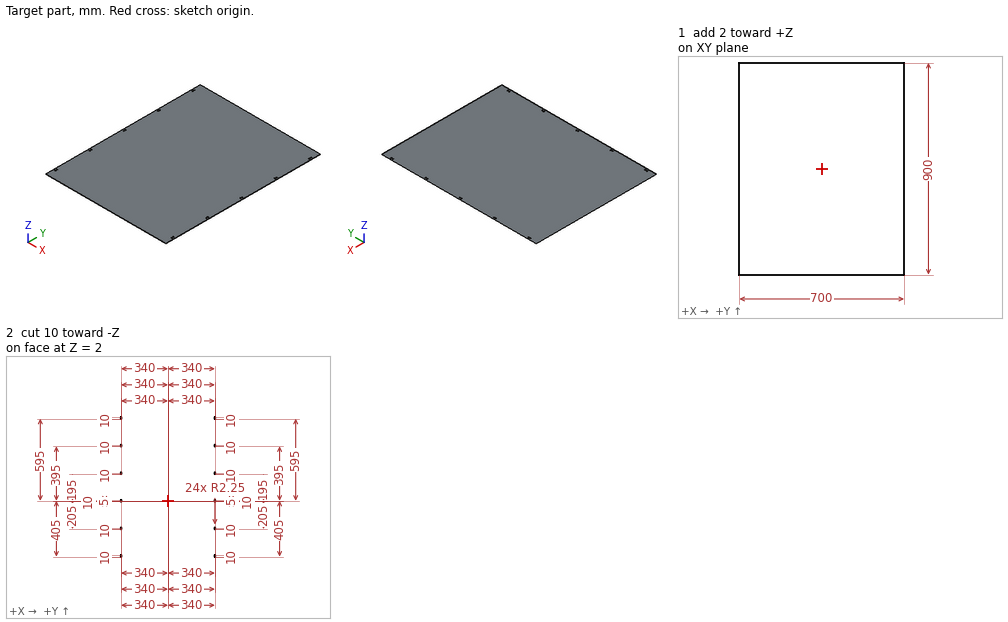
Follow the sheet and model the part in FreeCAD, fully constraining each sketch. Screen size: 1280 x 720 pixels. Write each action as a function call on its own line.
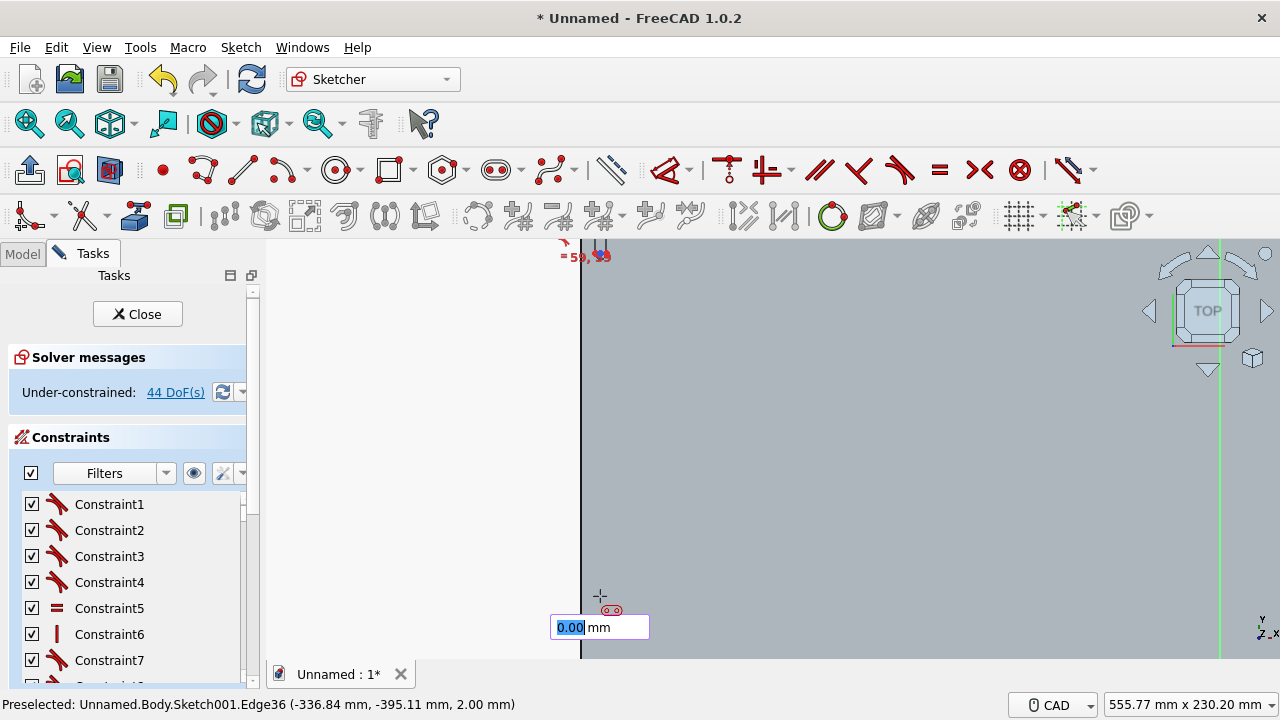
scroll(603, 606, up, 7)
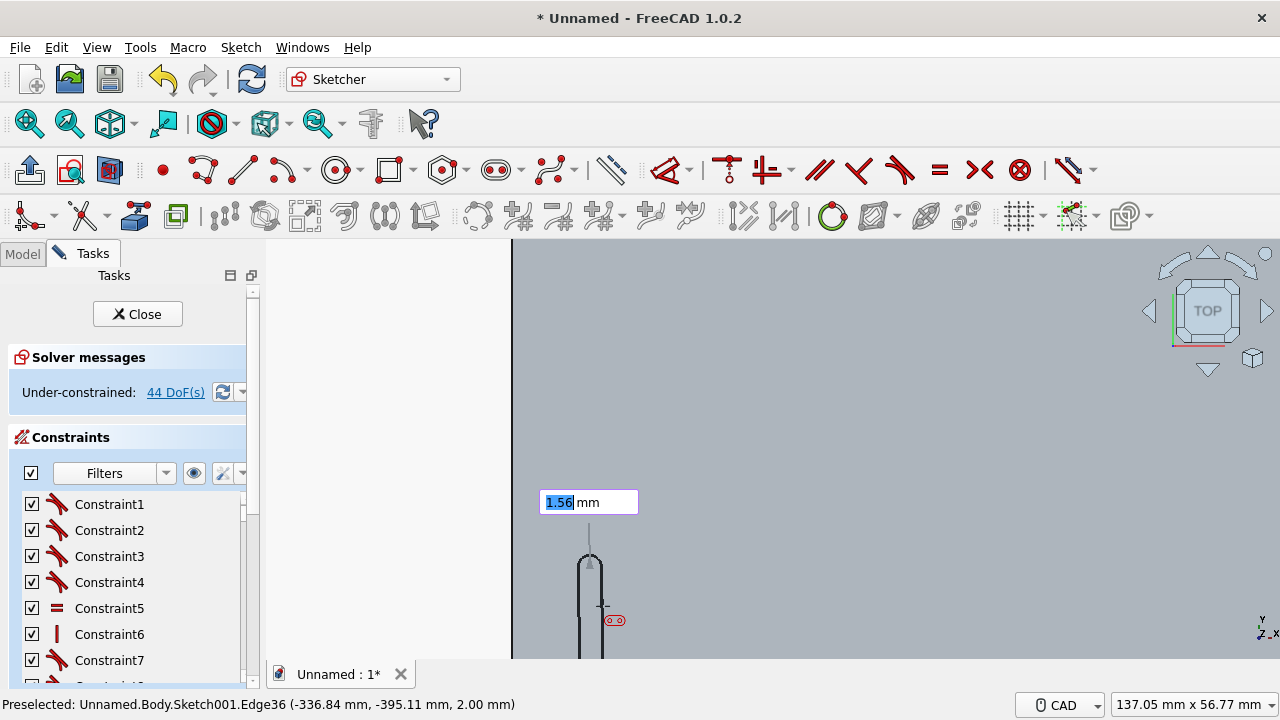
click(603, 601)
key(Escape)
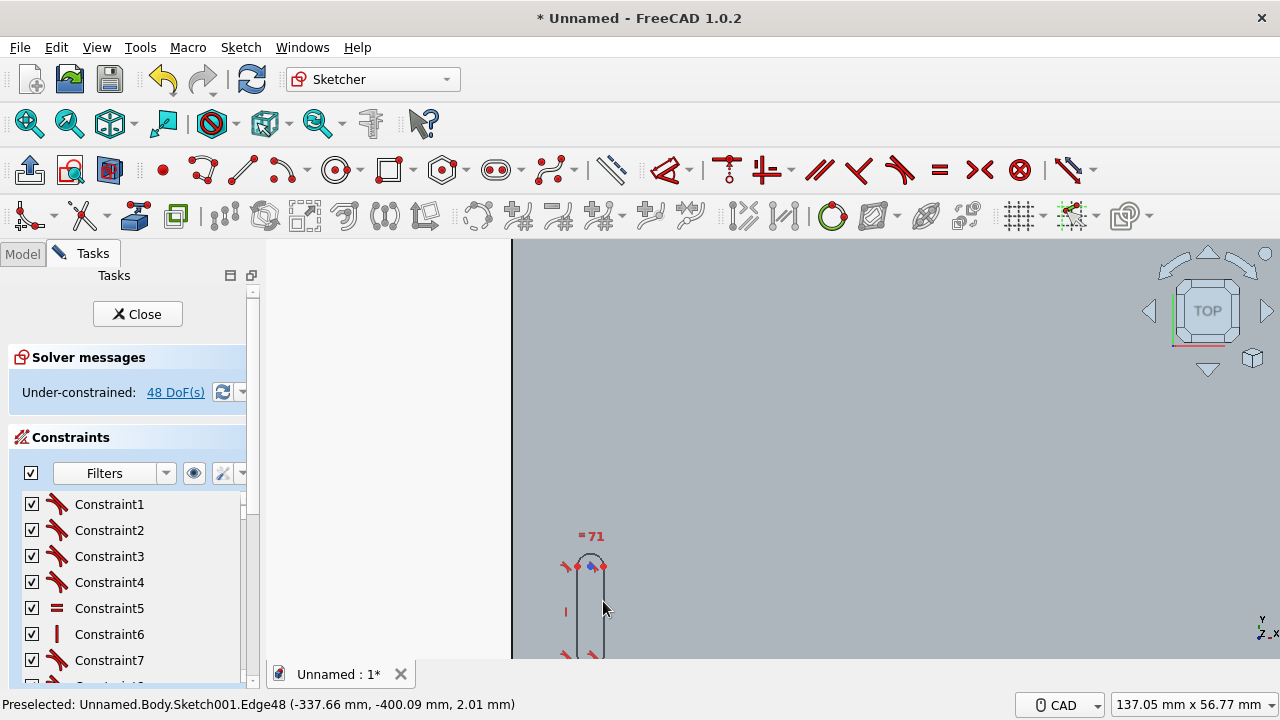
scroll(603, 600, down, 16)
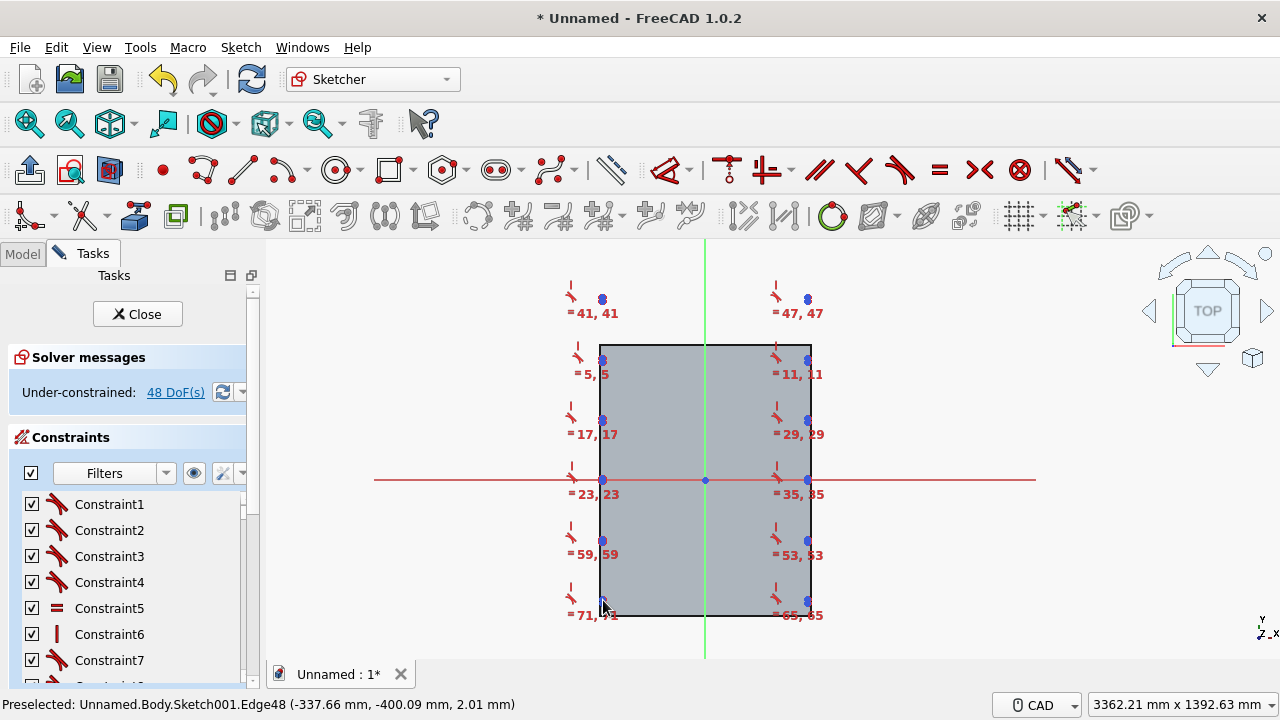
scroll(602, 363, up, 13)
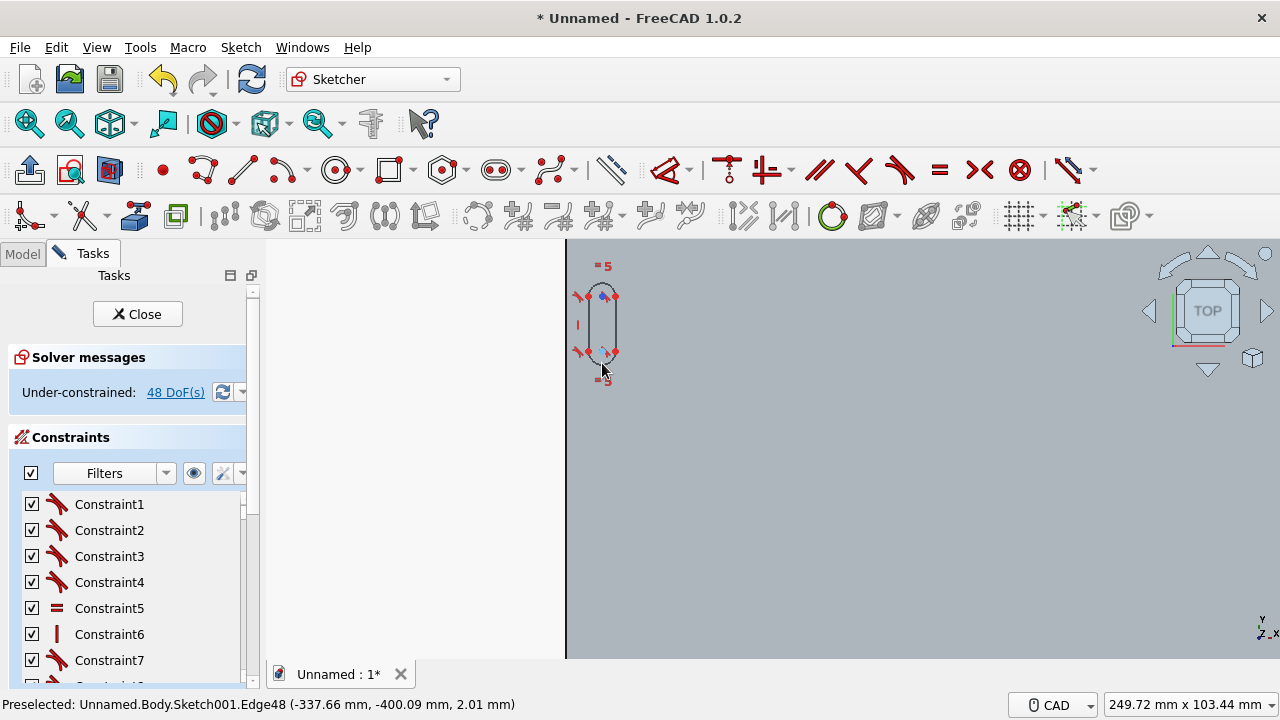
click(594, 362)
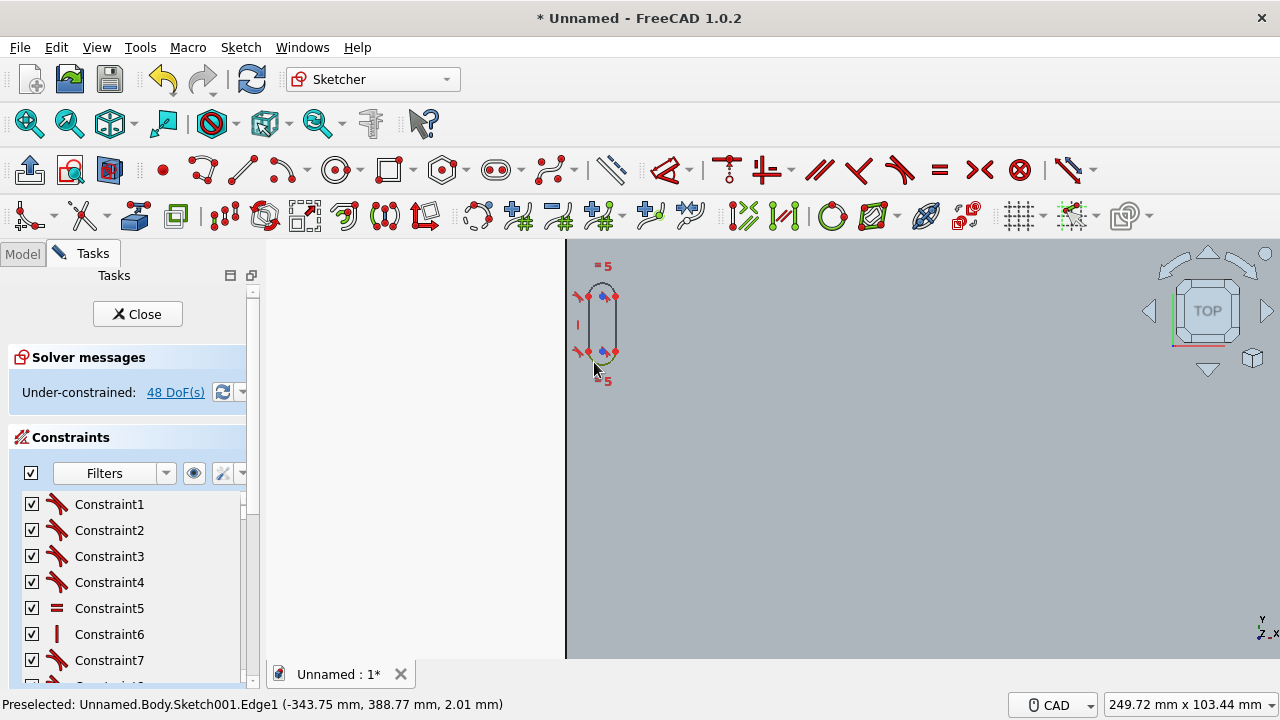
scroll(621, 379, down, 14)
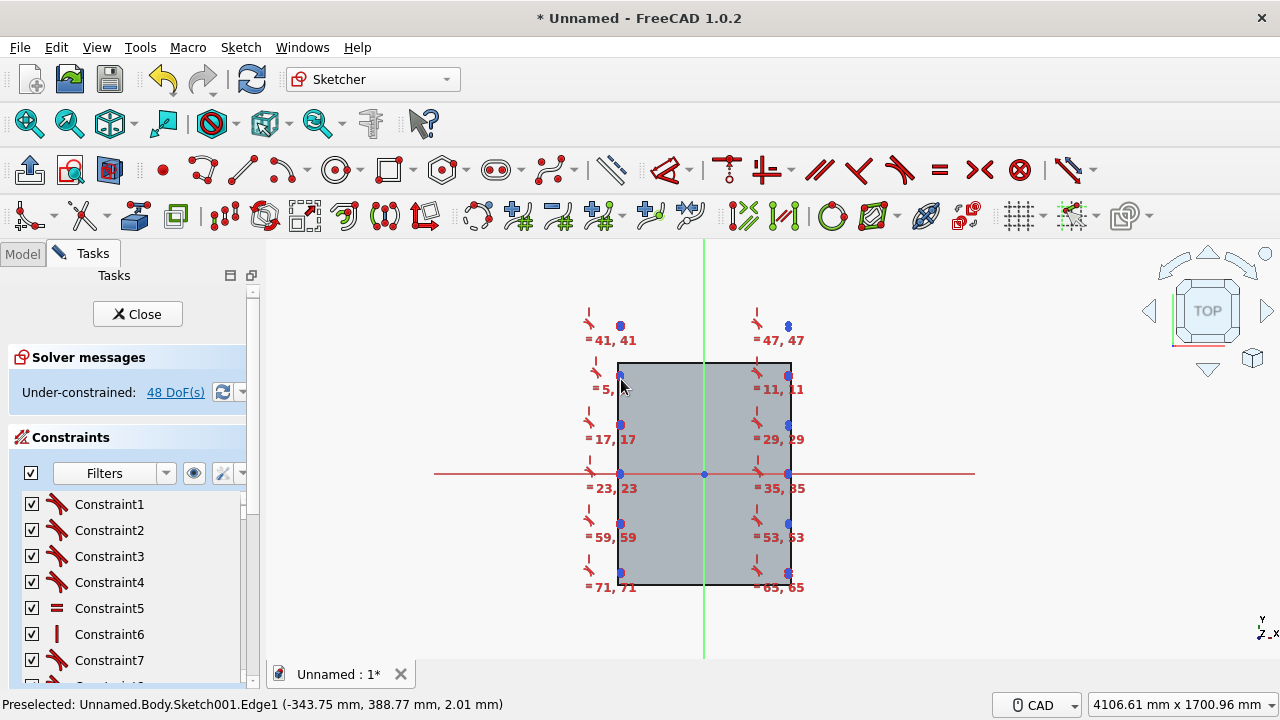
scroll(788, 378, up, 14)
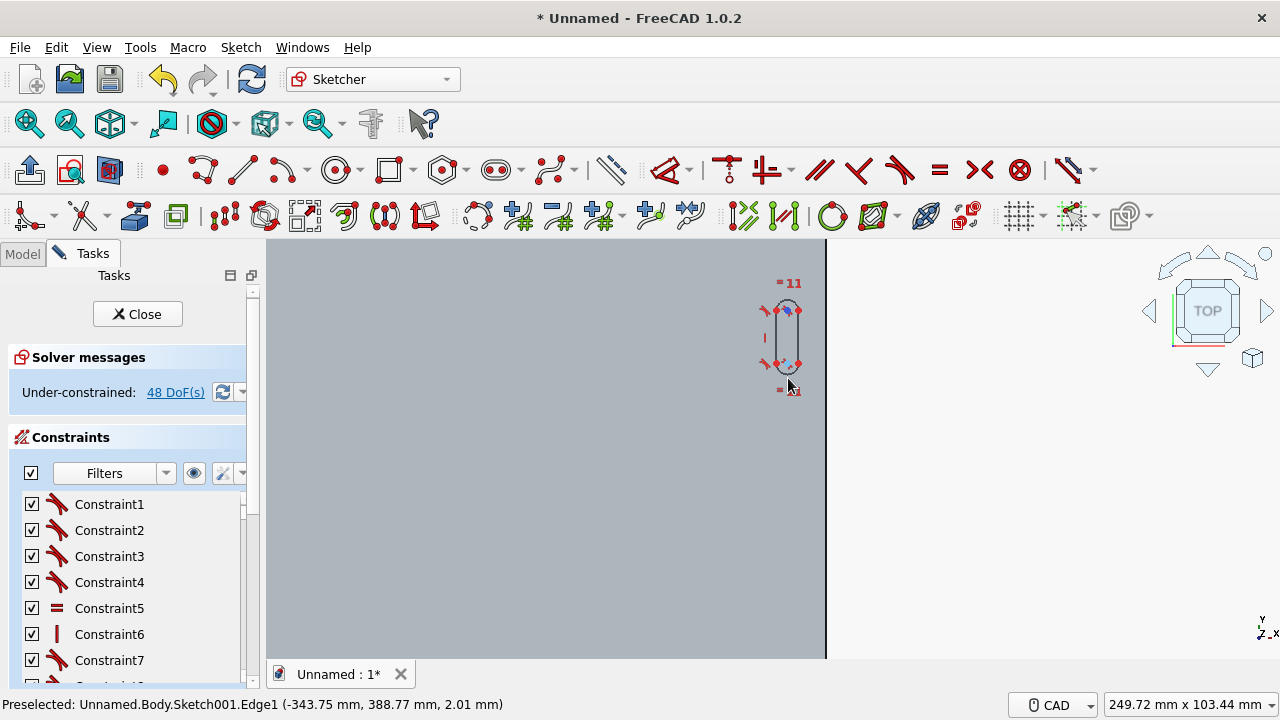
click(781, 372)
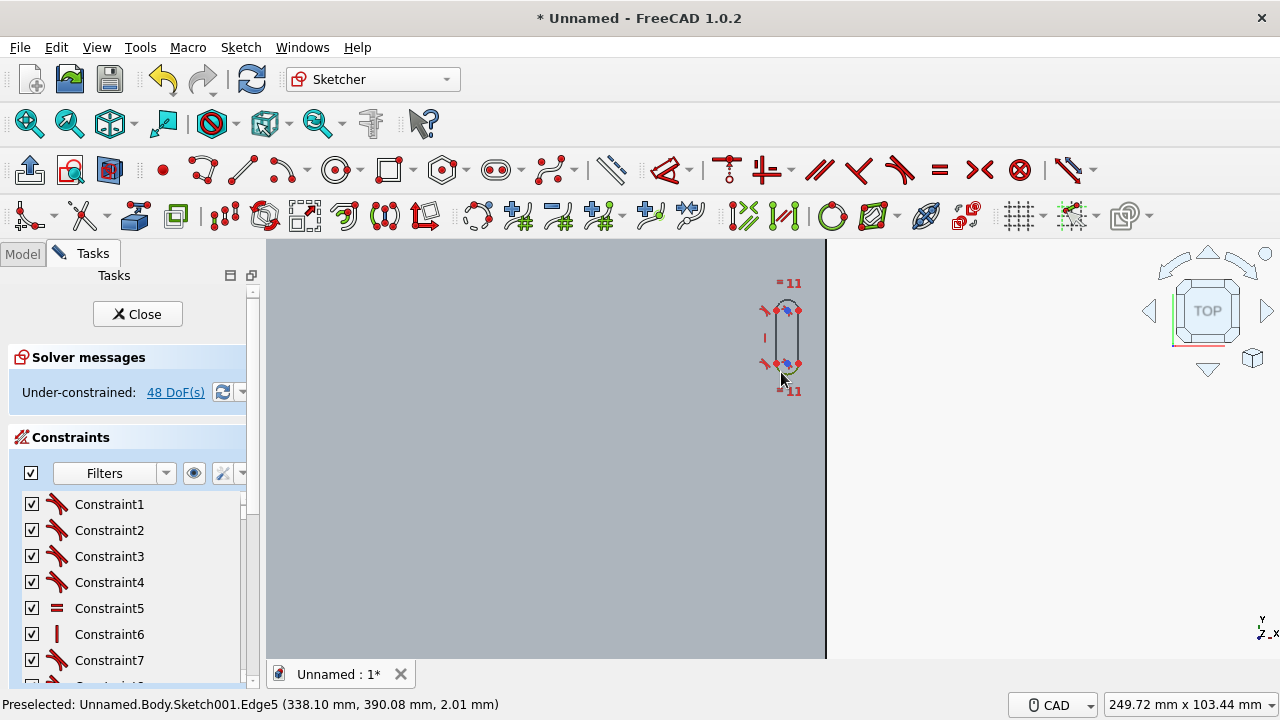
scroll(789, 378, down, 14)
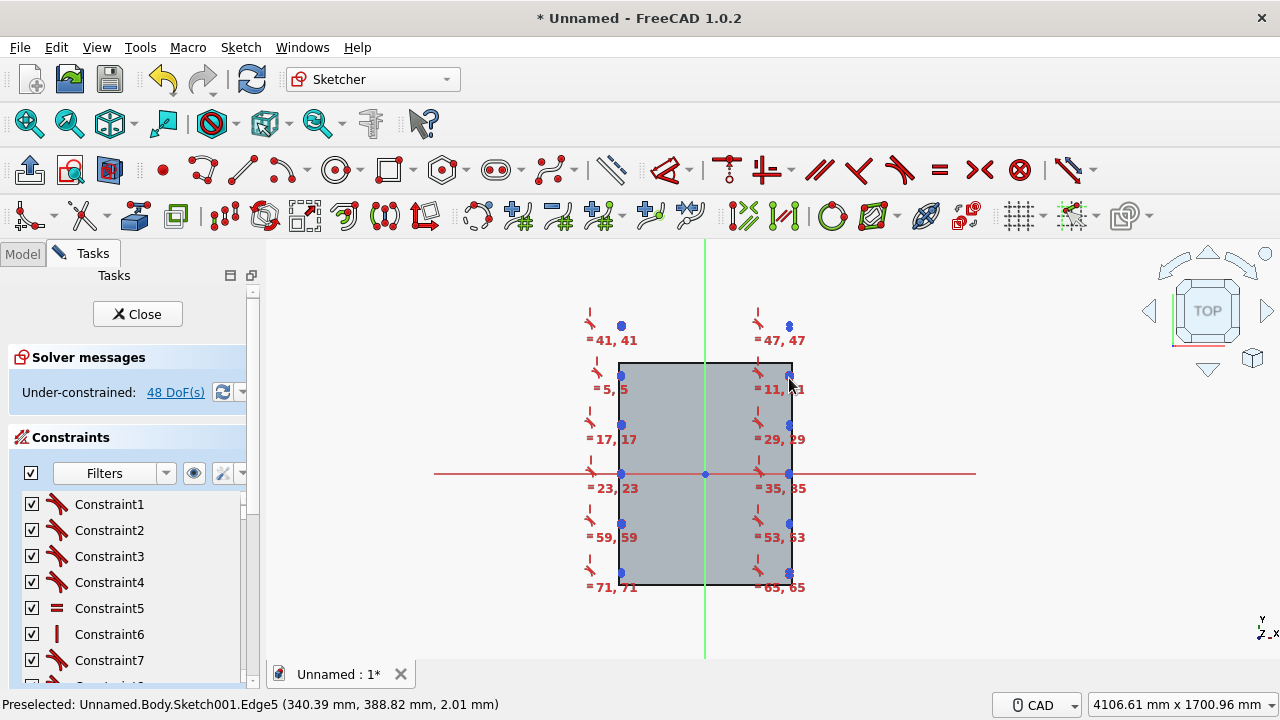
scroll(621, 427, up, 14)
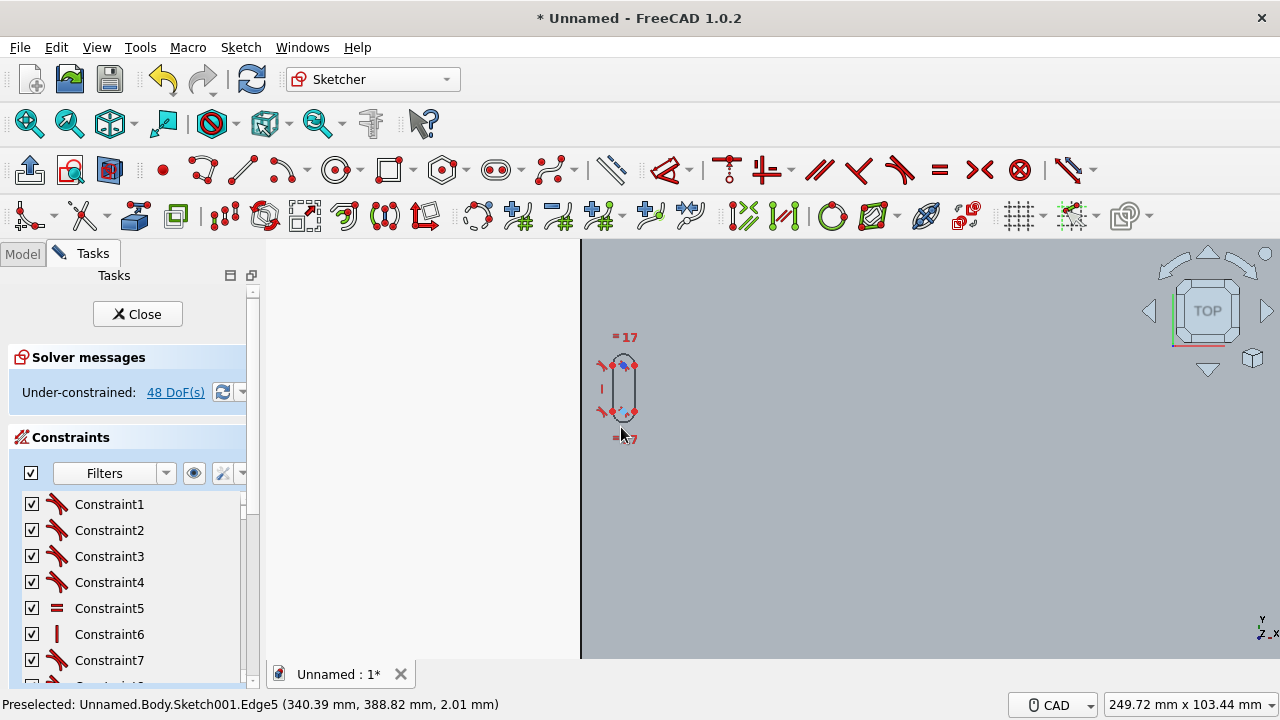
click(617, 420)